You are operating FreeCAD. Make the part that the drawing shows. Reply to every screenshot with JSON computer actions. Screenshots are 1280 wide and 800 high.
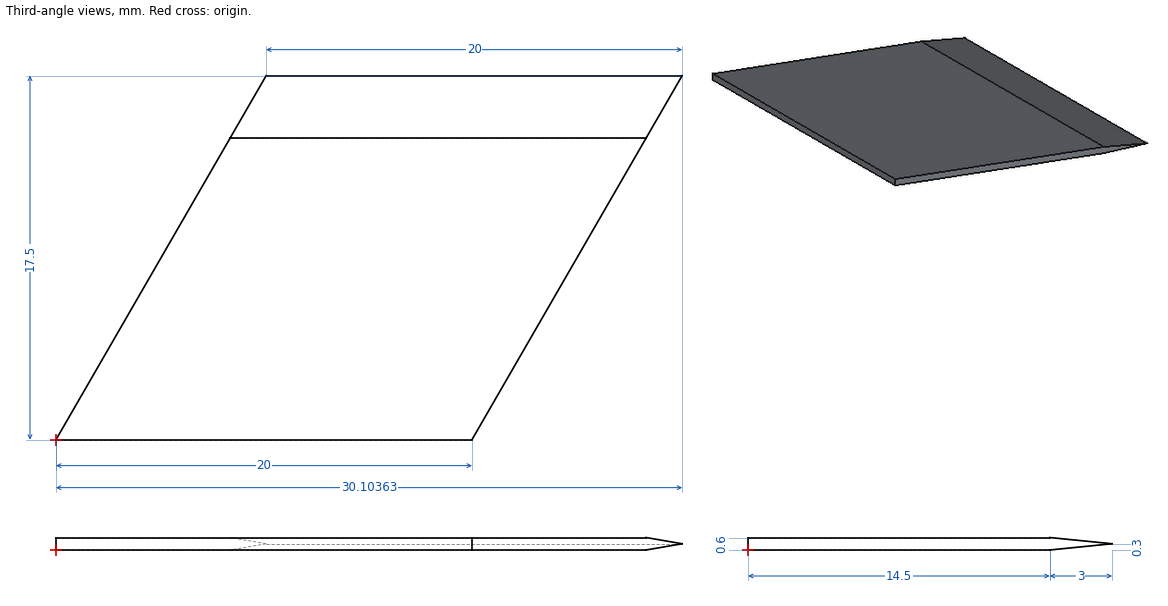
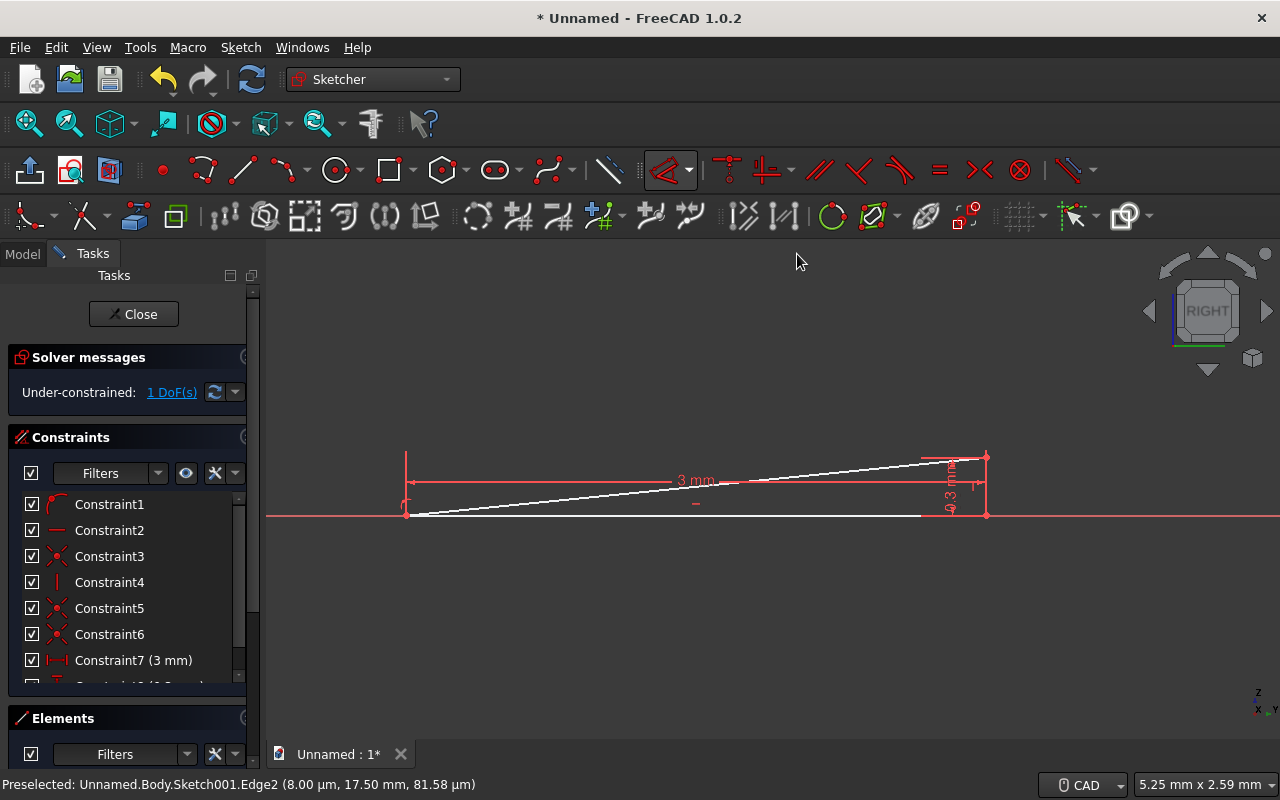
{"action": "left_click", "coordinate": [406, 516]}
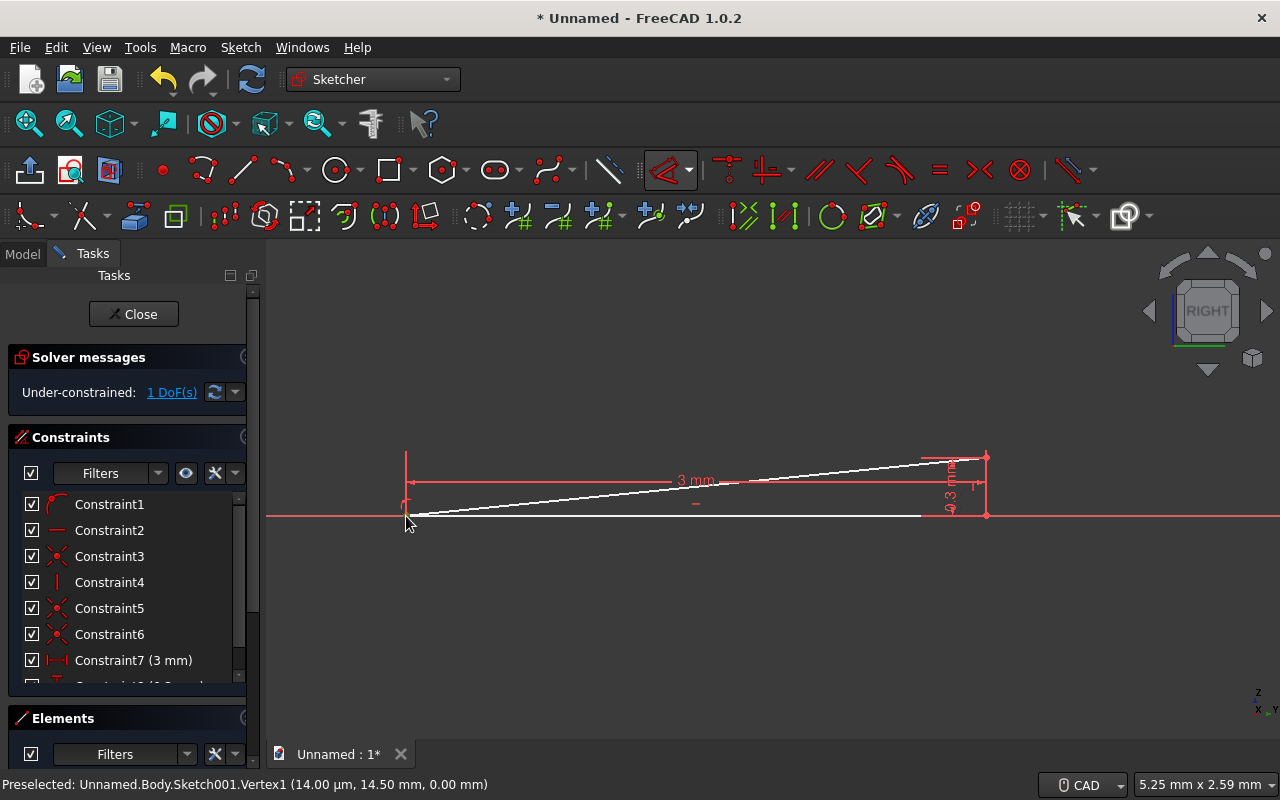
{"action": "key", "text": "l"}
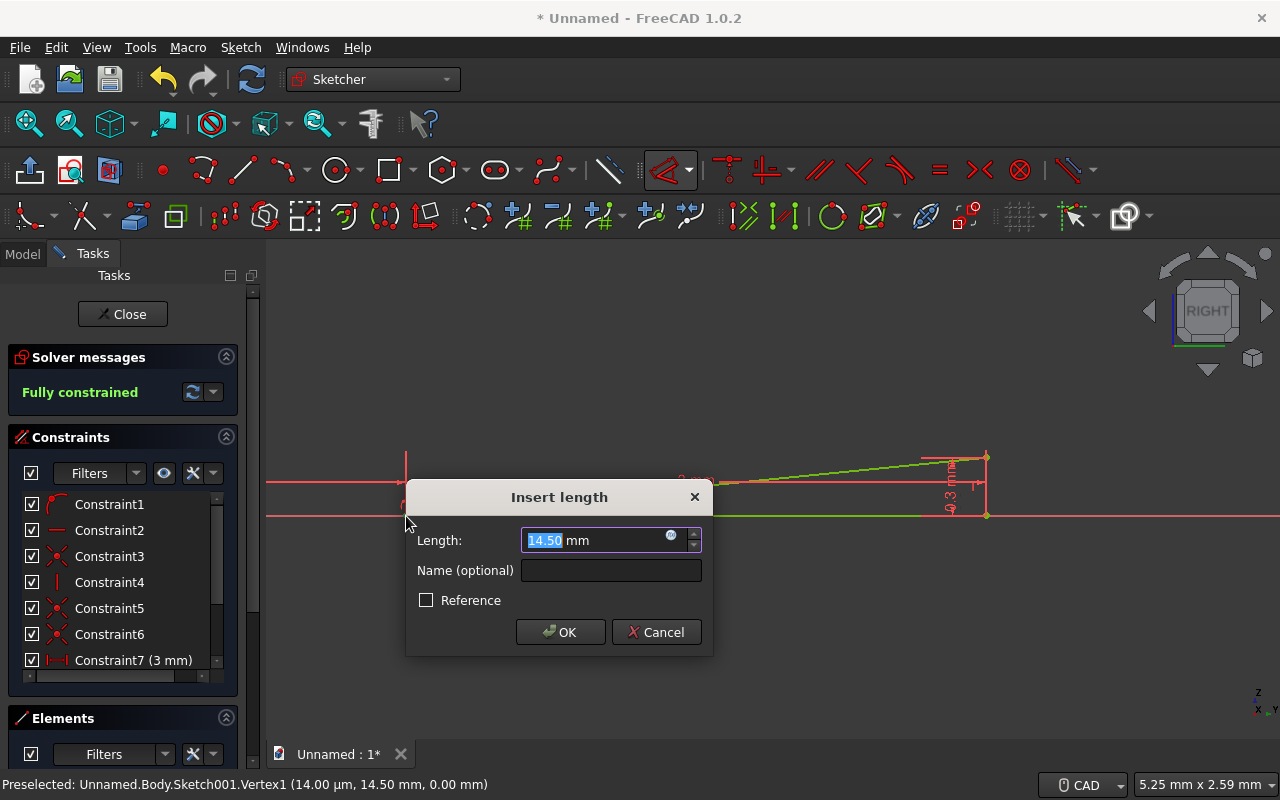
{"action": "type", "text": "14.5"}
{"action": "key", "text": "Return"}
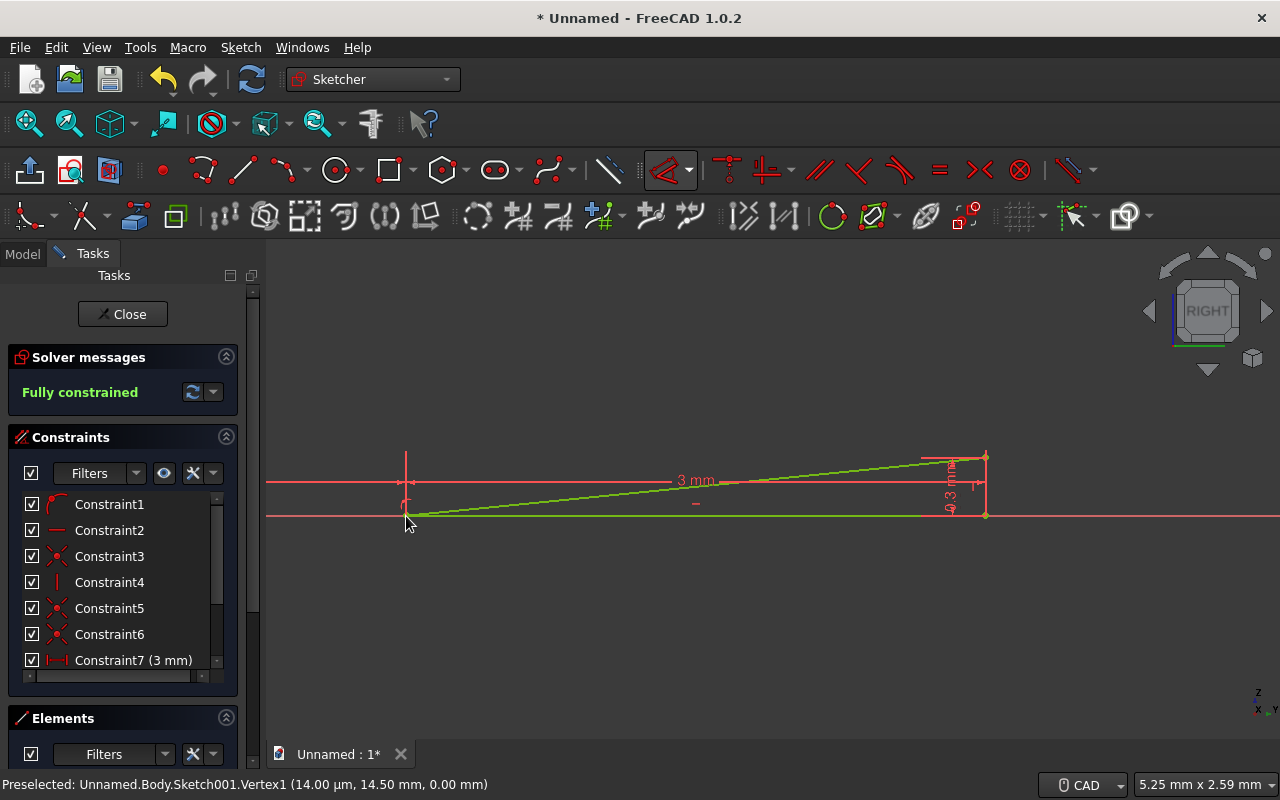
{"action": "left_click", "coordinate": [123, 314]}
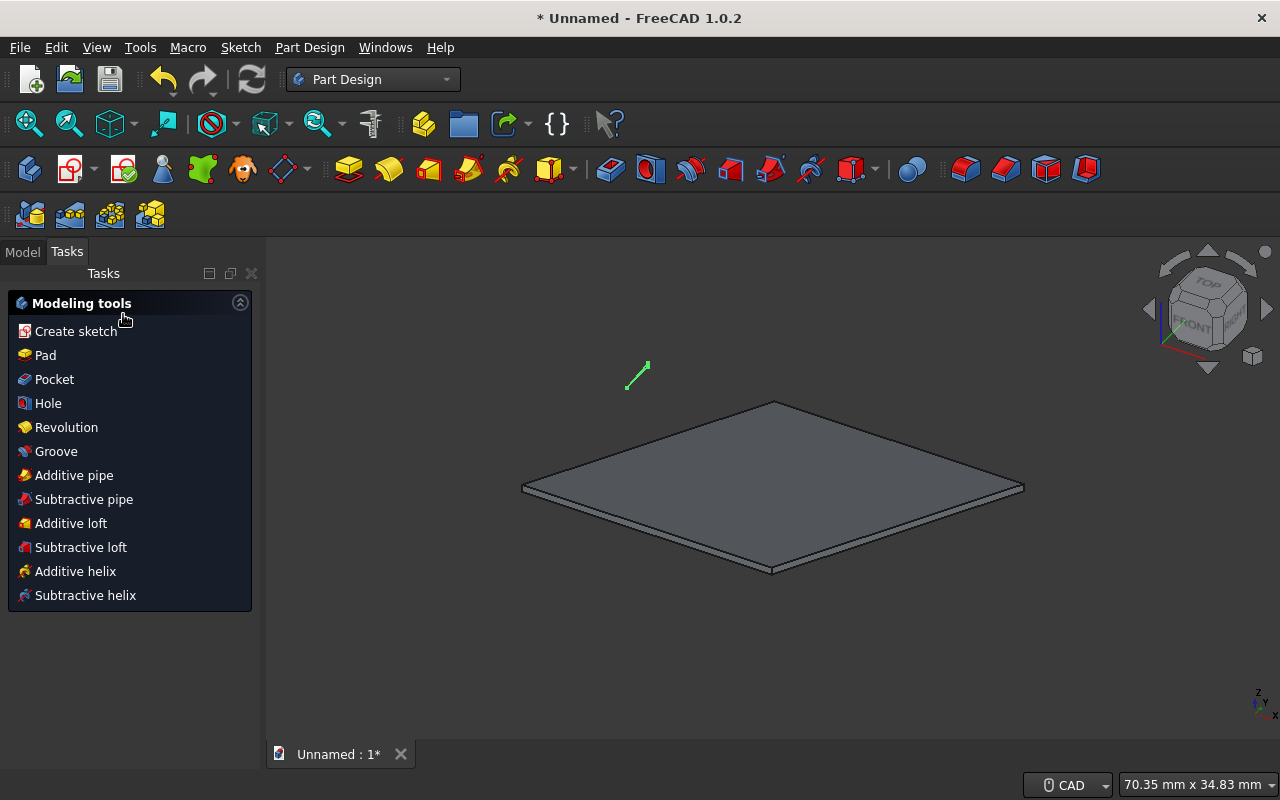
{"action": "left_click", "coordinate": [612, 170]}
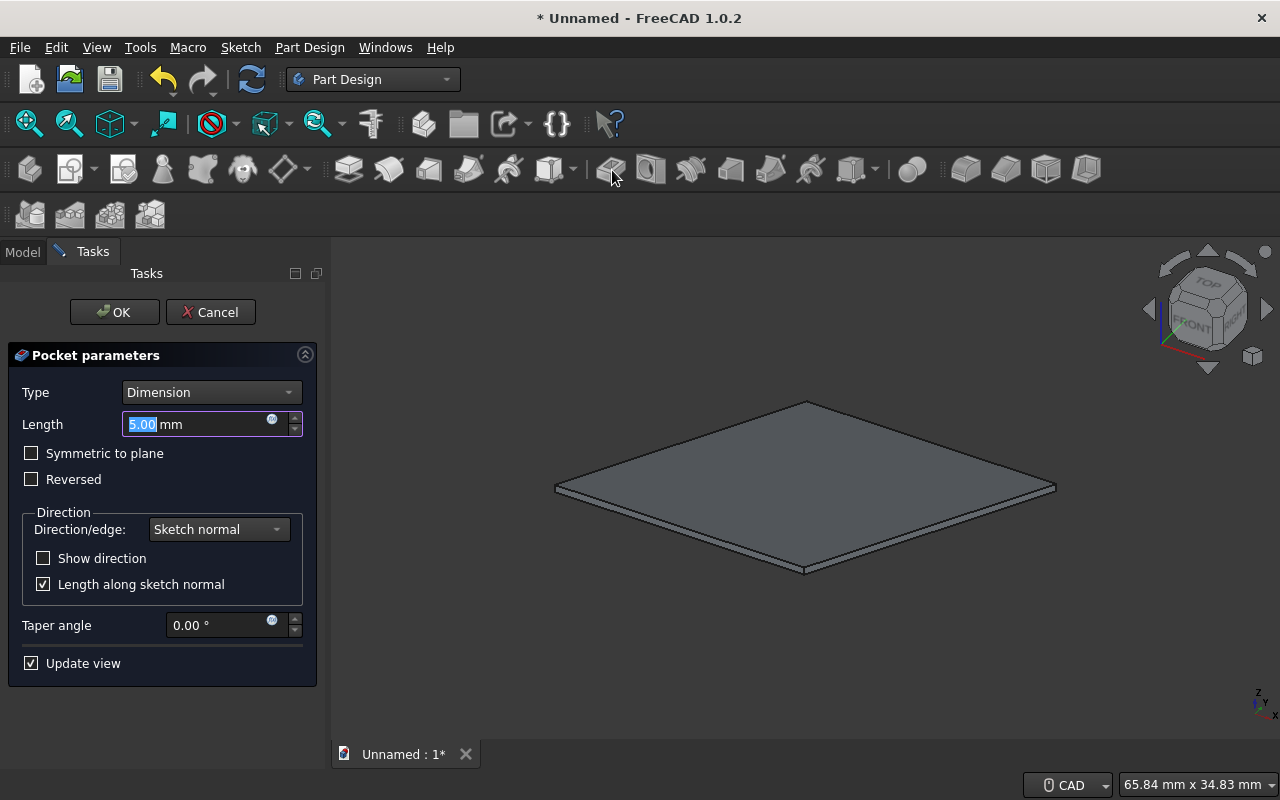
{"action": "left_click", "coordinate": [212, 392]}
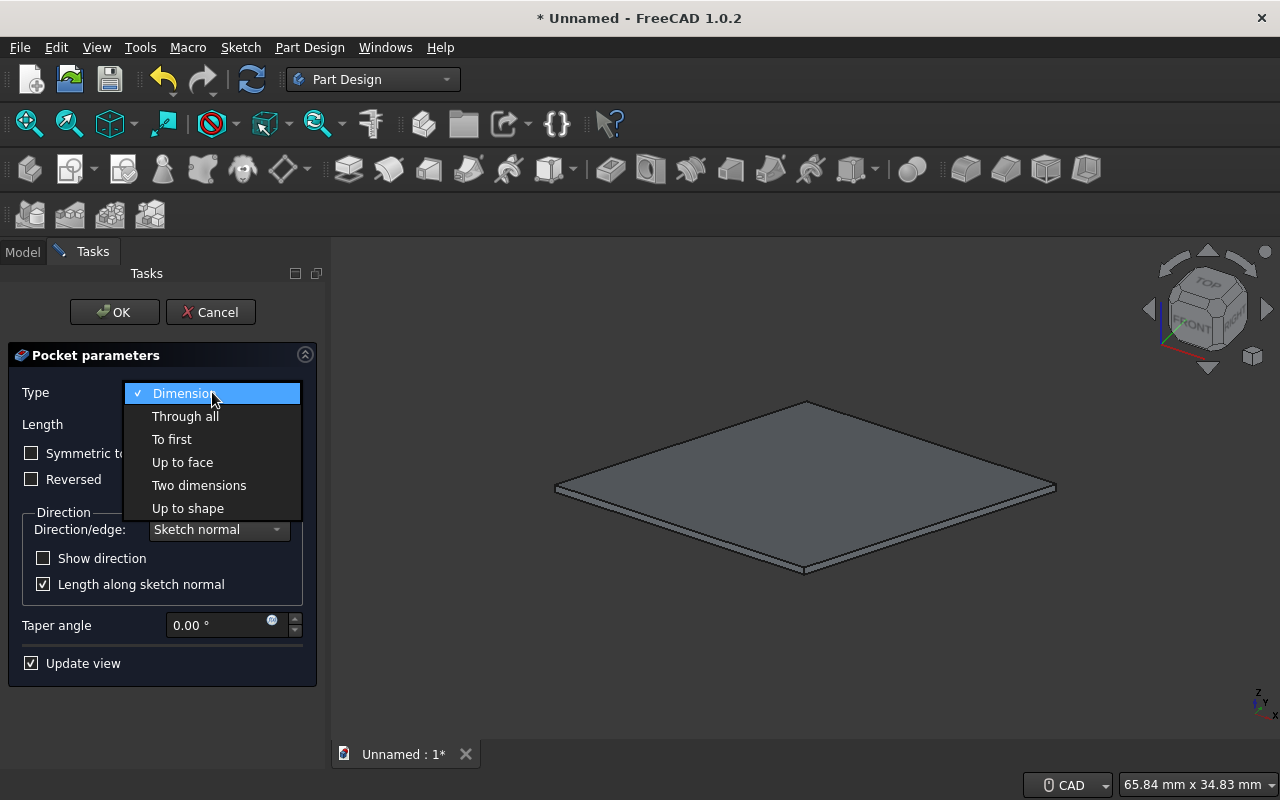
{"action": "left_click", "coordinate": [212, 416]}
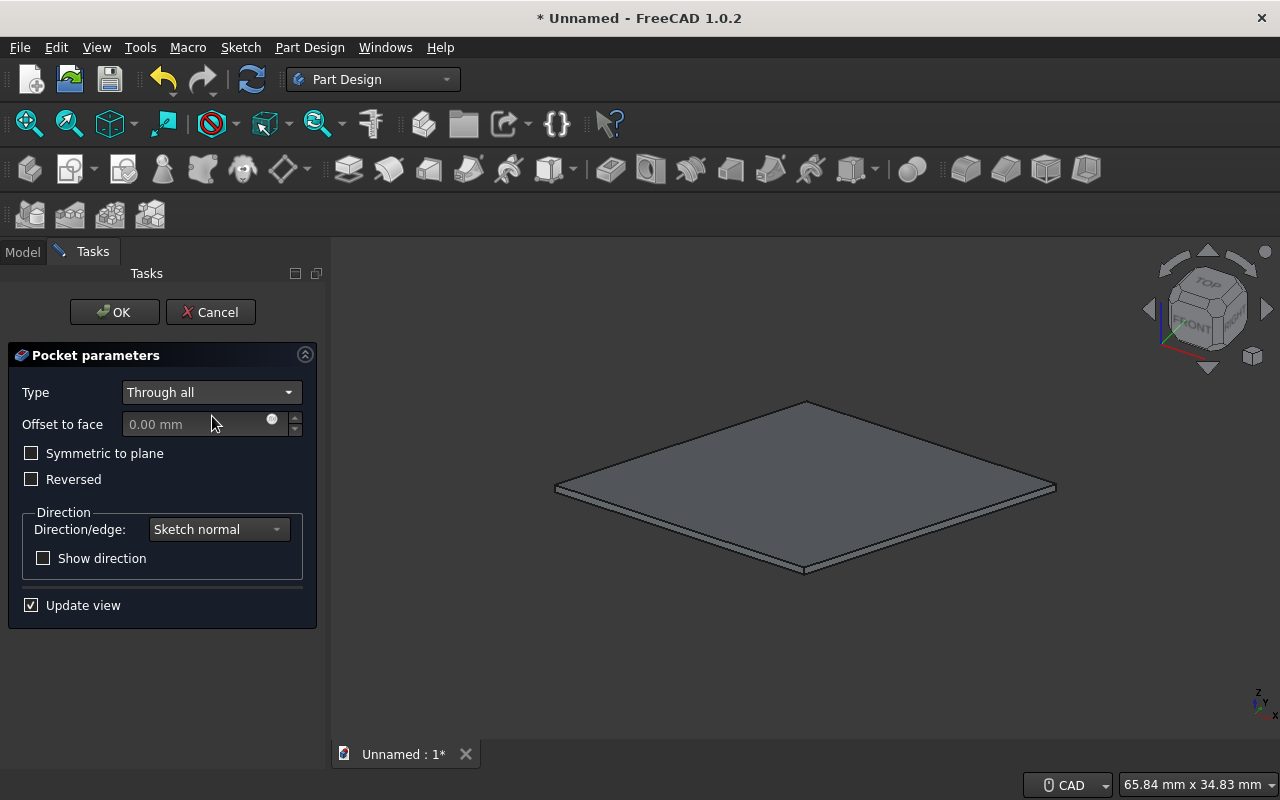
{"action": "left_click", "coordinate": [30, 479]}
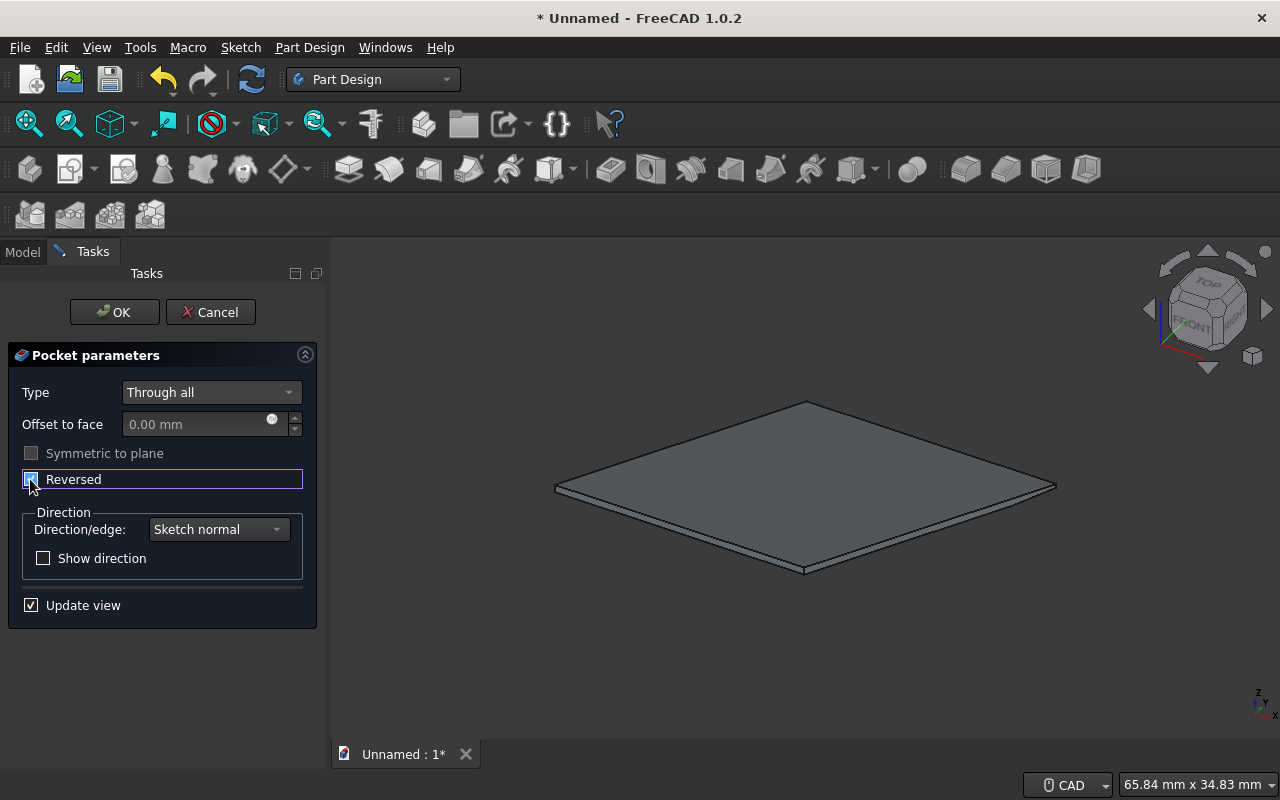
{"action": "left_click", "coordinate": [115, 312]}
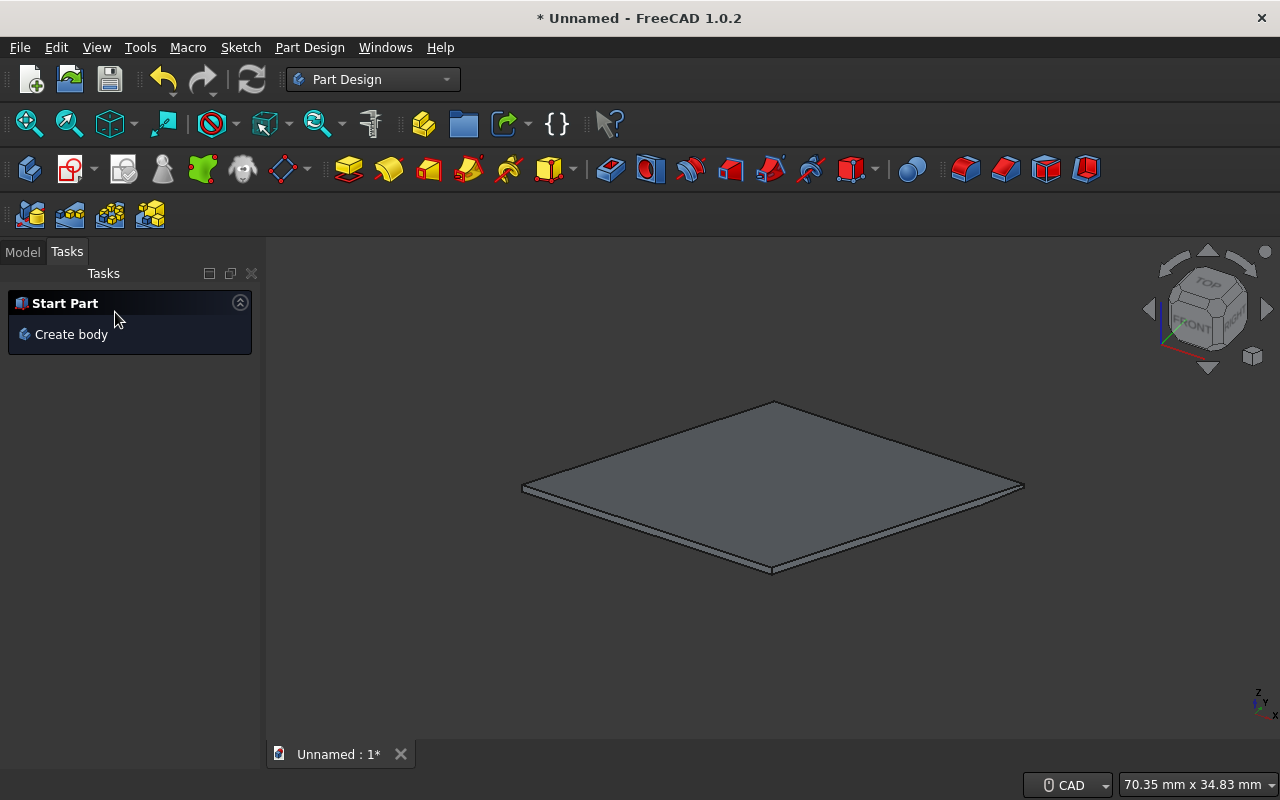
{"action": "left_click", "coordinate": [23, 251]}